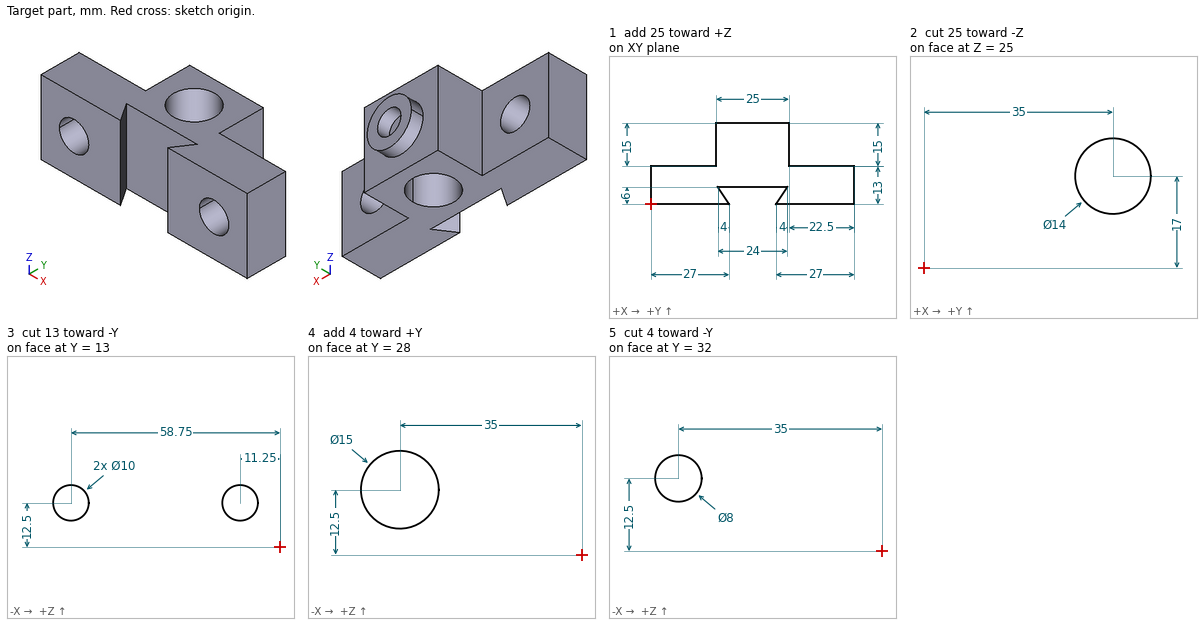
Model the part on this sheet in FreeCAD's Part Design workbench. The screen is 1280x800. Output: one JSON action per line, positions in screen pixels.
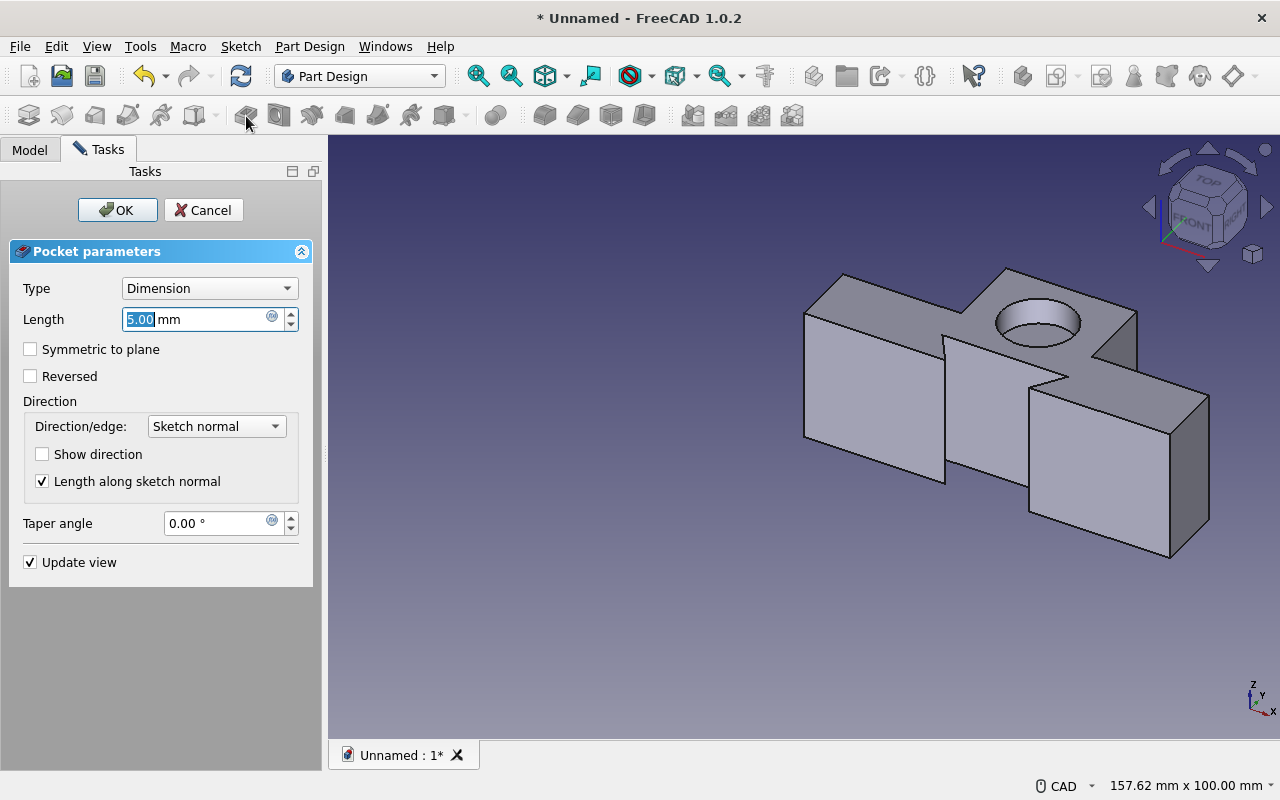
{"action": "type", "text": "25"}
{"action": "key", "text": "Tab"}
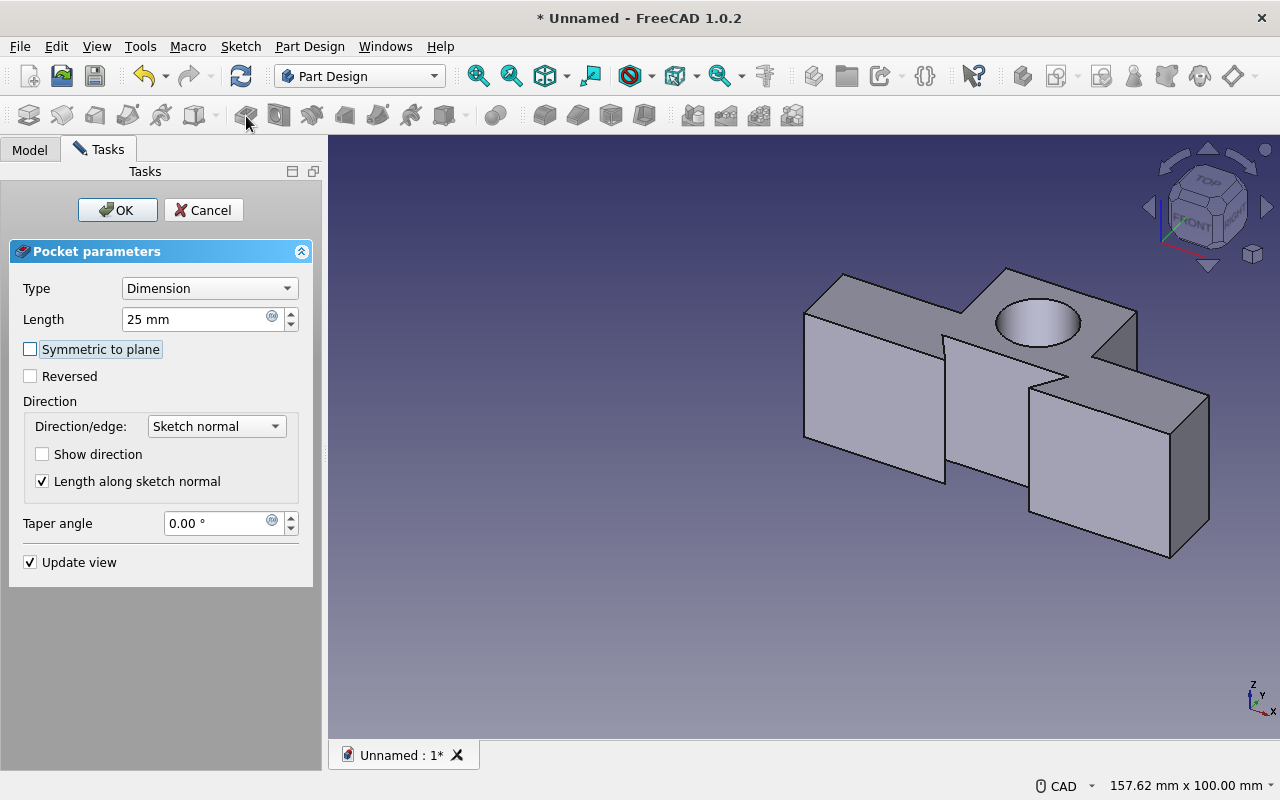
{"action": "left_click", "coordinate": [118, 210]}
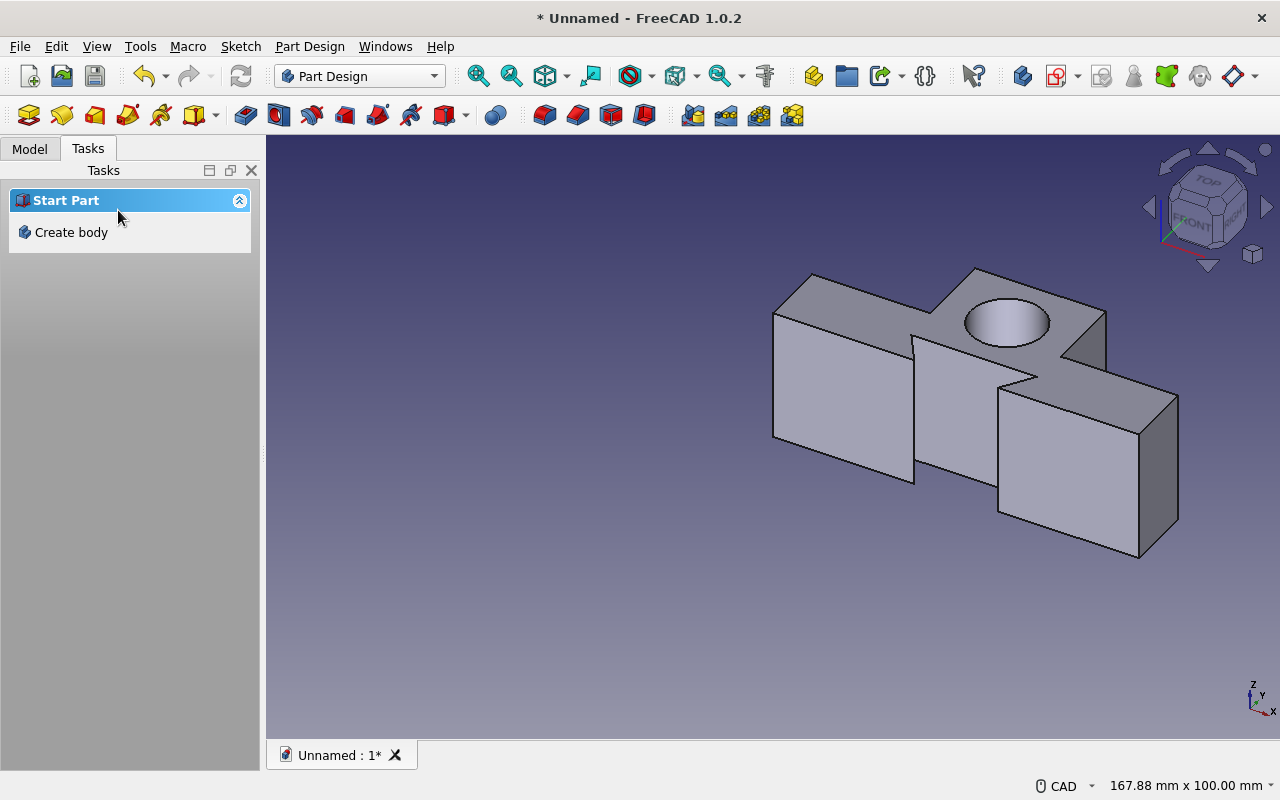
{"action": "key", "text": "4"}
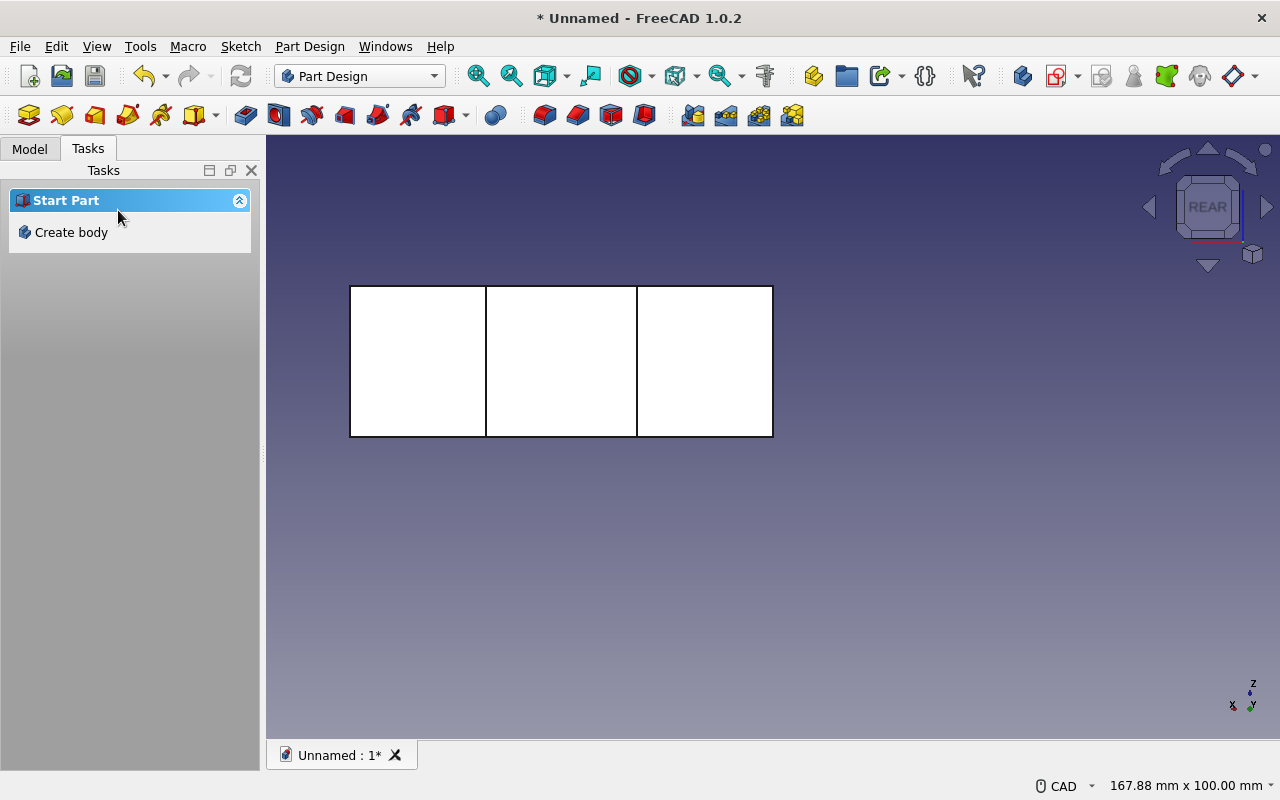
{"action": "left_click", "coordinate": [479, 76]}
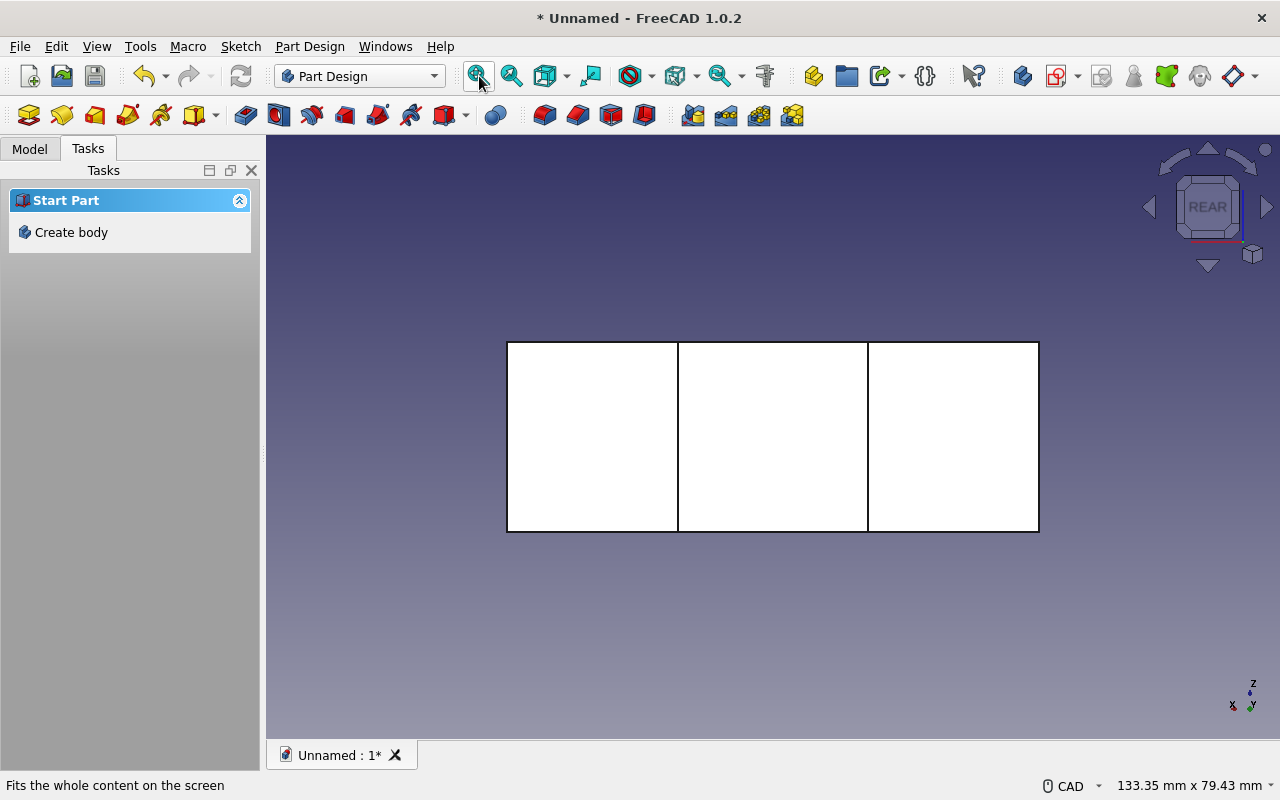
{"action": "left_click", "coordinate": [954, 436]}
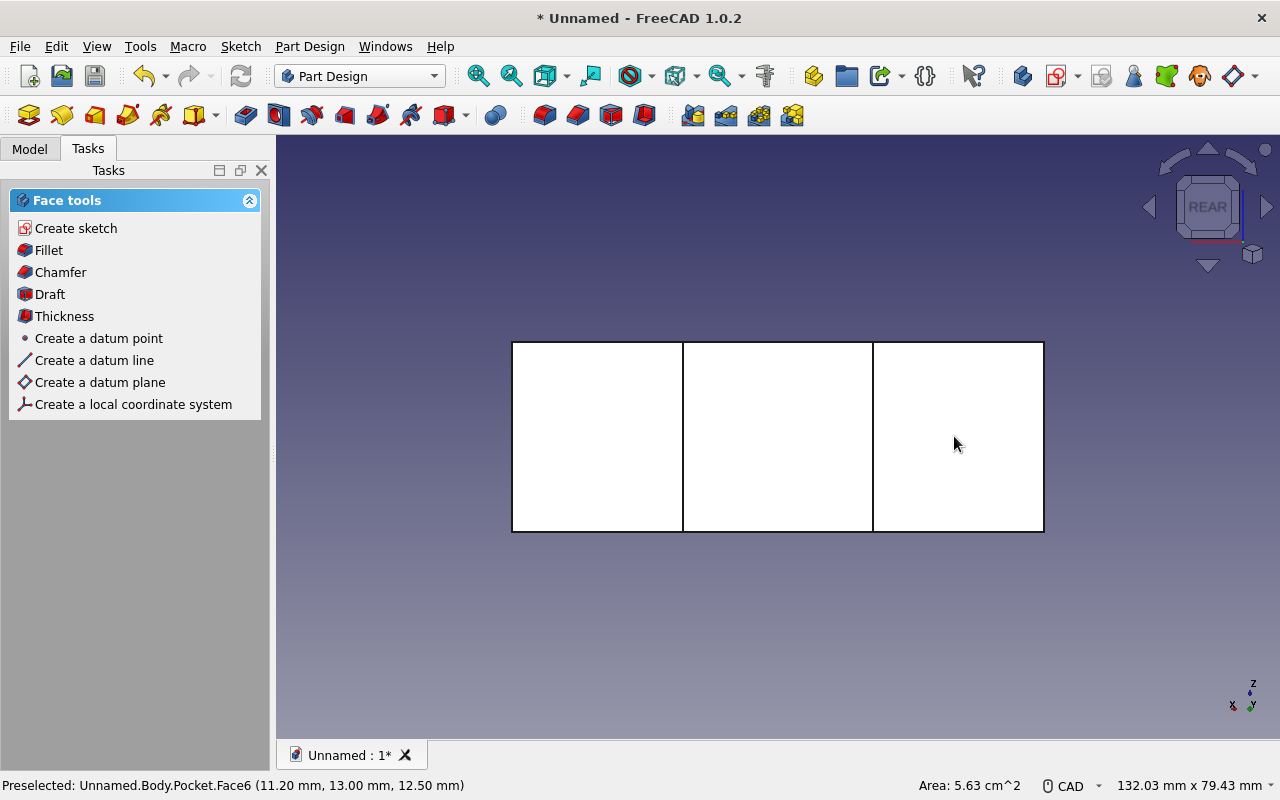
{"action": "left_click", "coordinate": [1056, 76]}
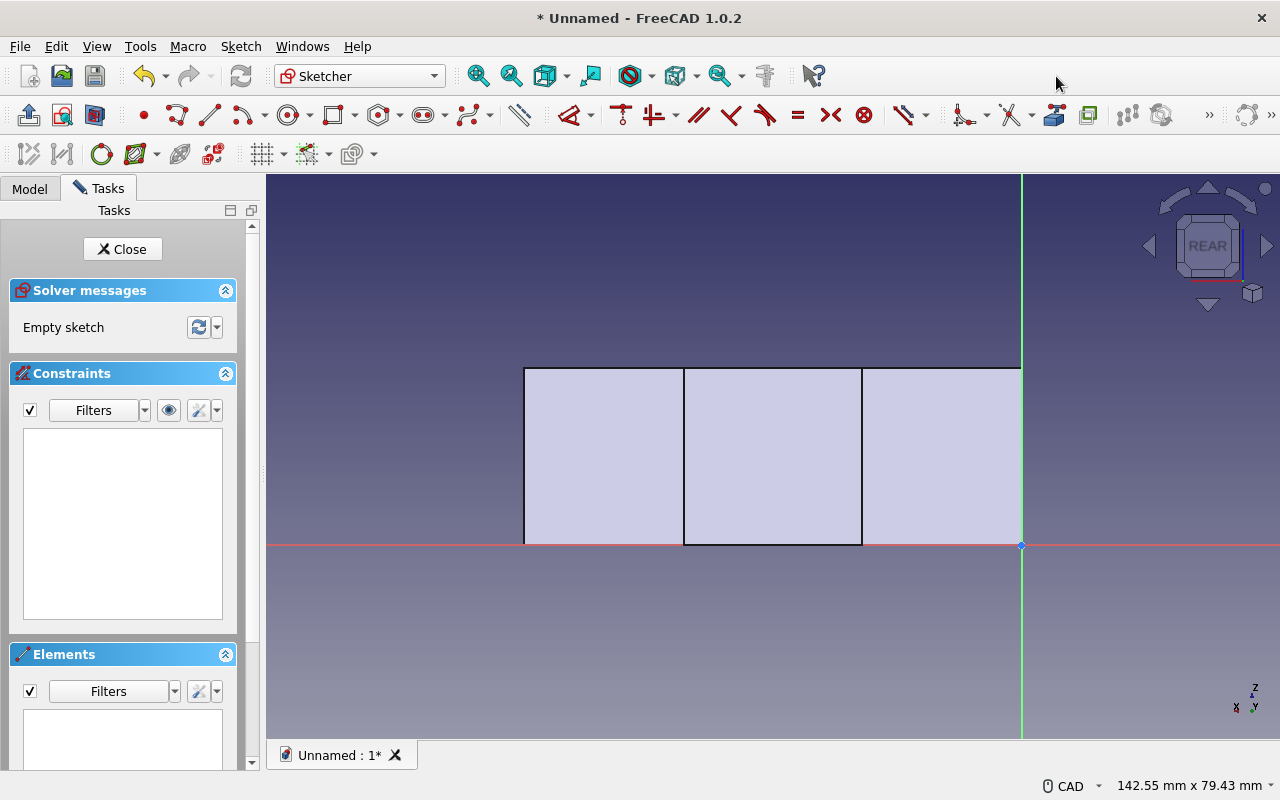
{"action": "left_click", "coordinate": [288, 116]}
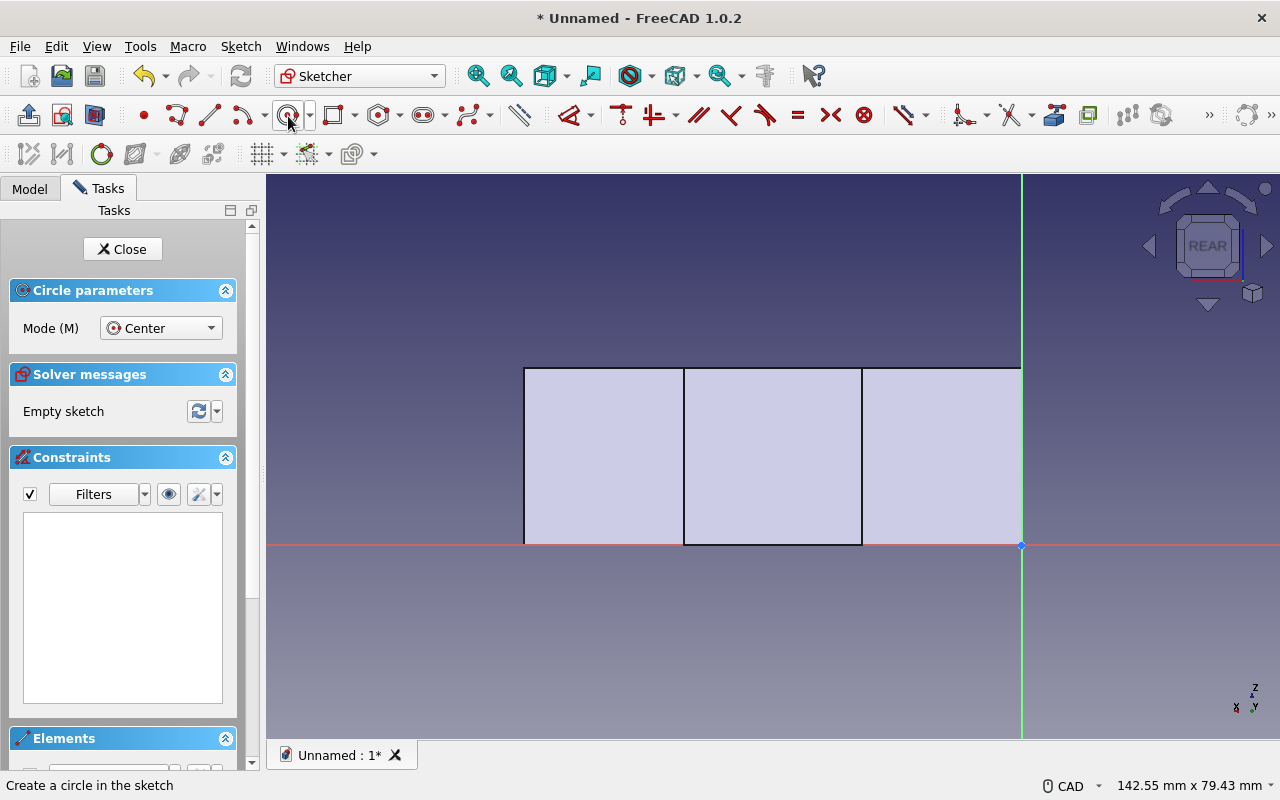
{"action": "left_click", "coordinate": [604, 456]}
{"action": "mouse_move", "coordinate": [629, 431]}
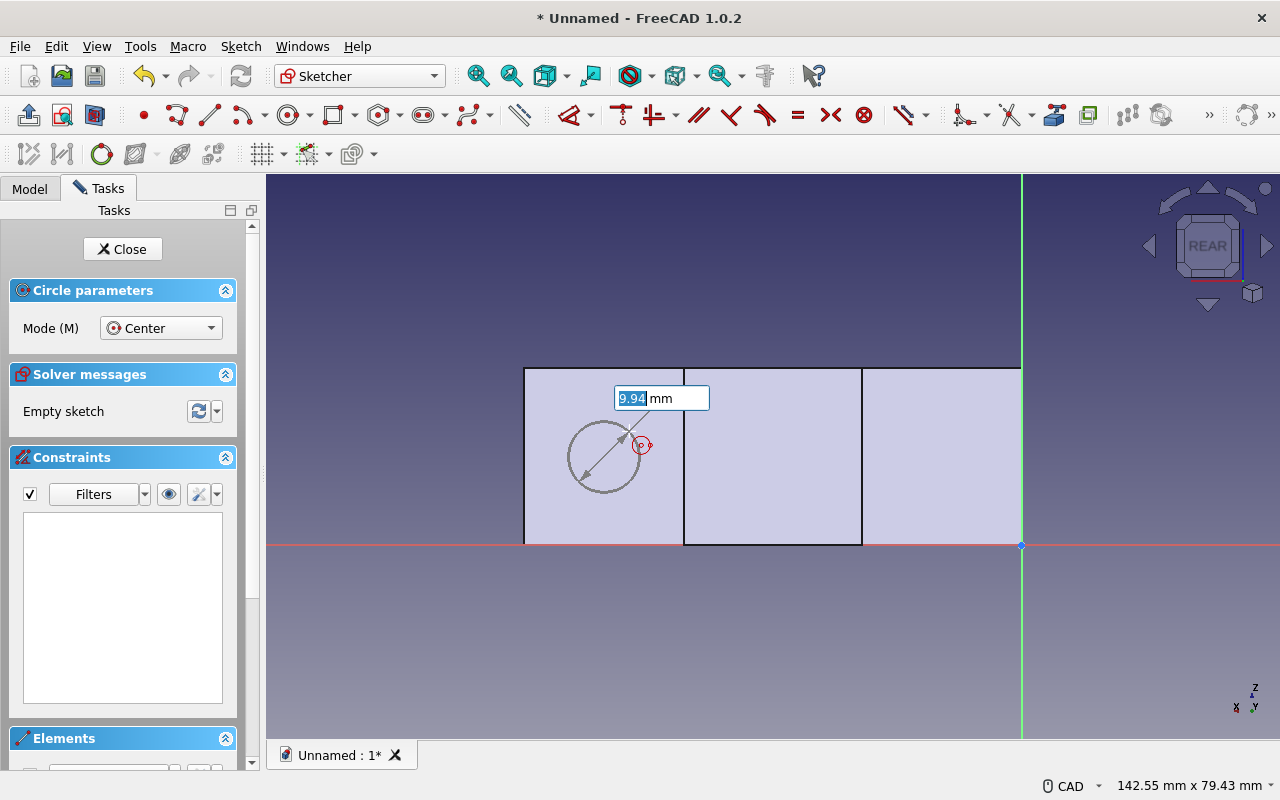
{"action": "type", "text": "10"}
{"action": "key", "text": "Return"}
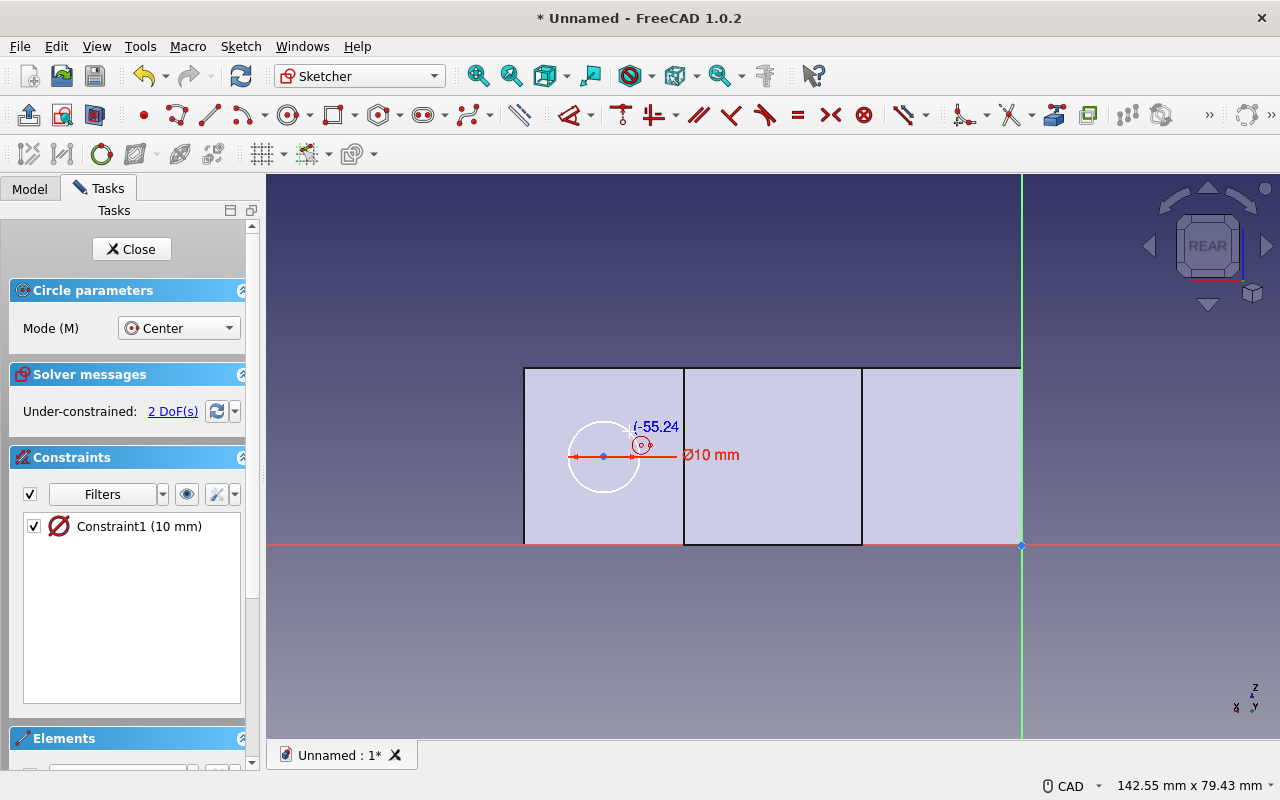
{"action": "left_click", "coordinate": [942, 456]}
{"action": "mouse_move", "coordinate": [967, 431]}